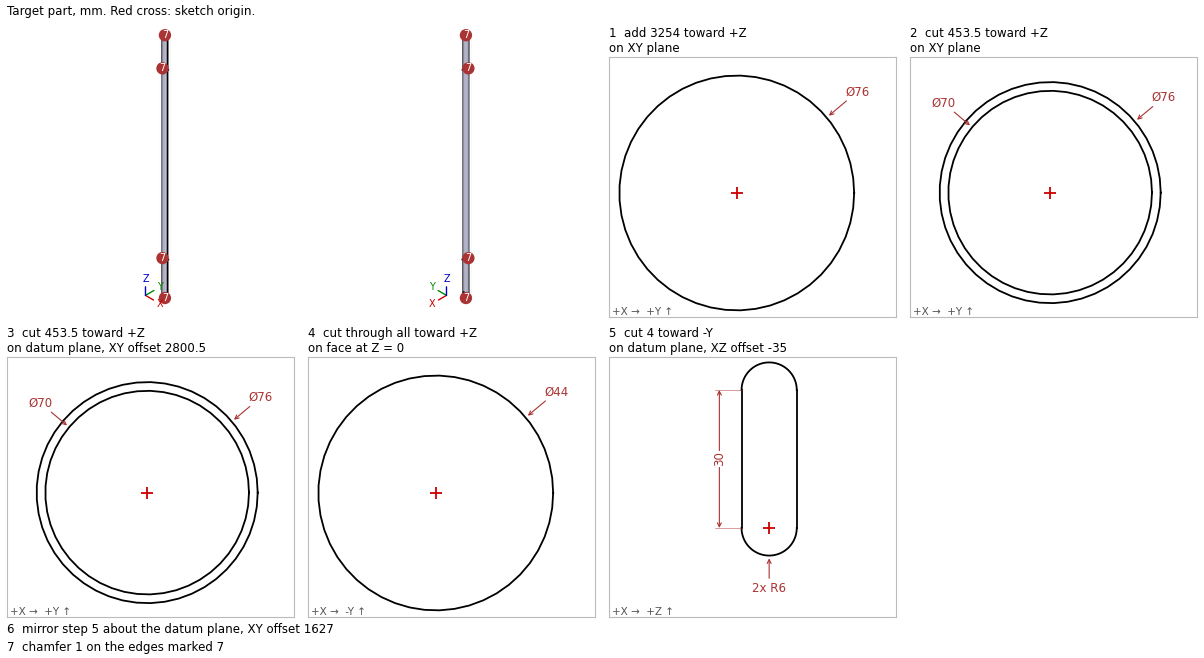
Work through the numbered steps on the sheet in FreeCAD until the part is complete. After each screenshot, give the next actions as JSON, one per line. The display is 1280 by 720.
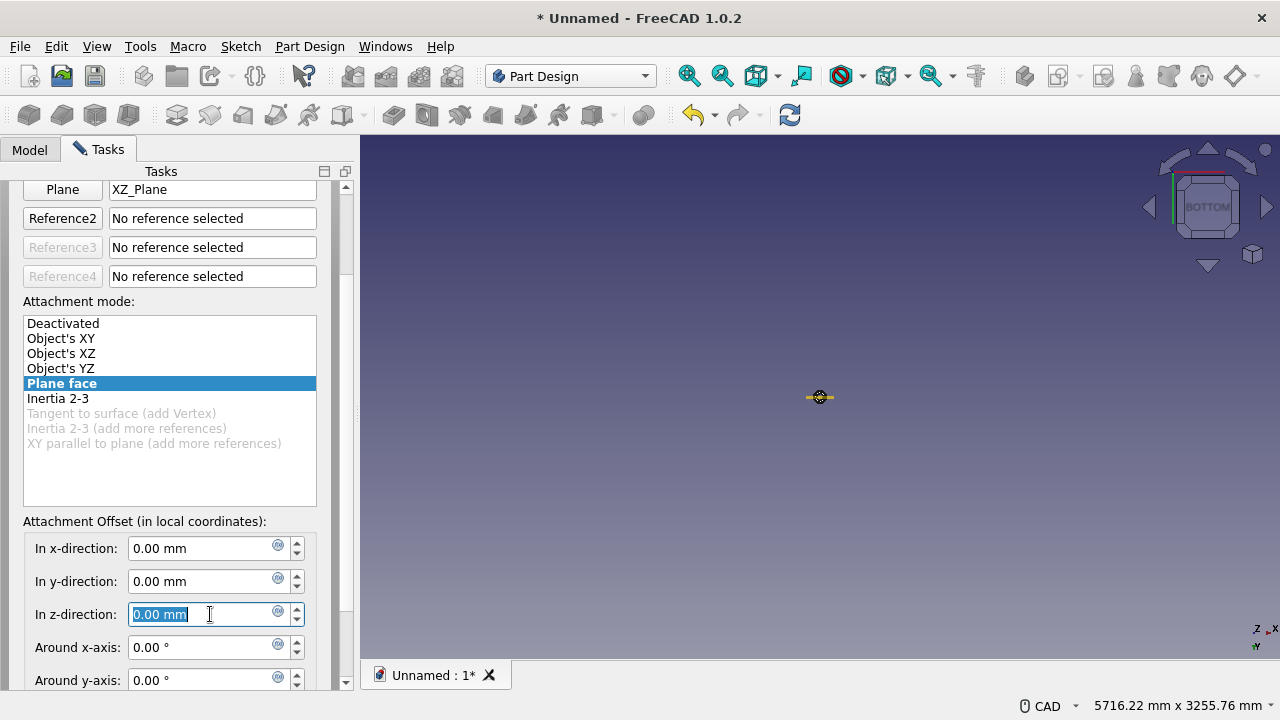
{"action": "type", "text": "-35"}
{"action": "key", "text": "Tab"}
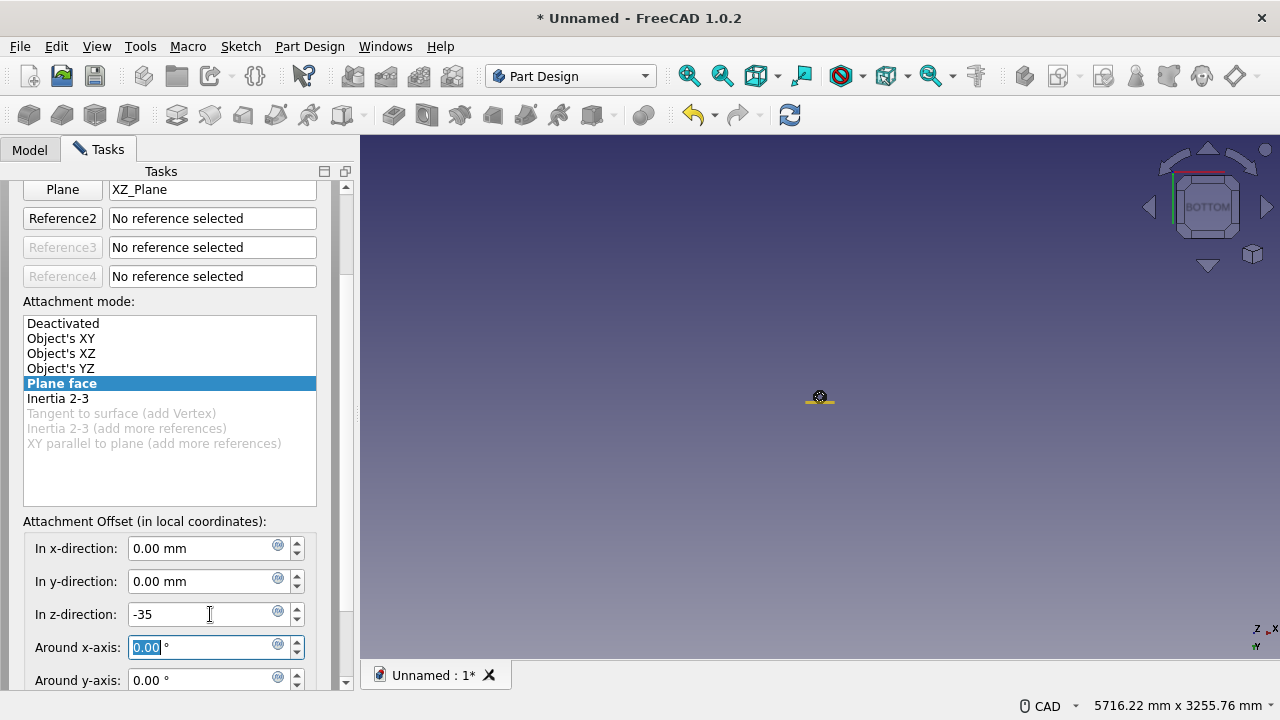
{"action": "scroll", "coordinate": [346, 436], "scroll_direction": "up", "scroll_amount": 3}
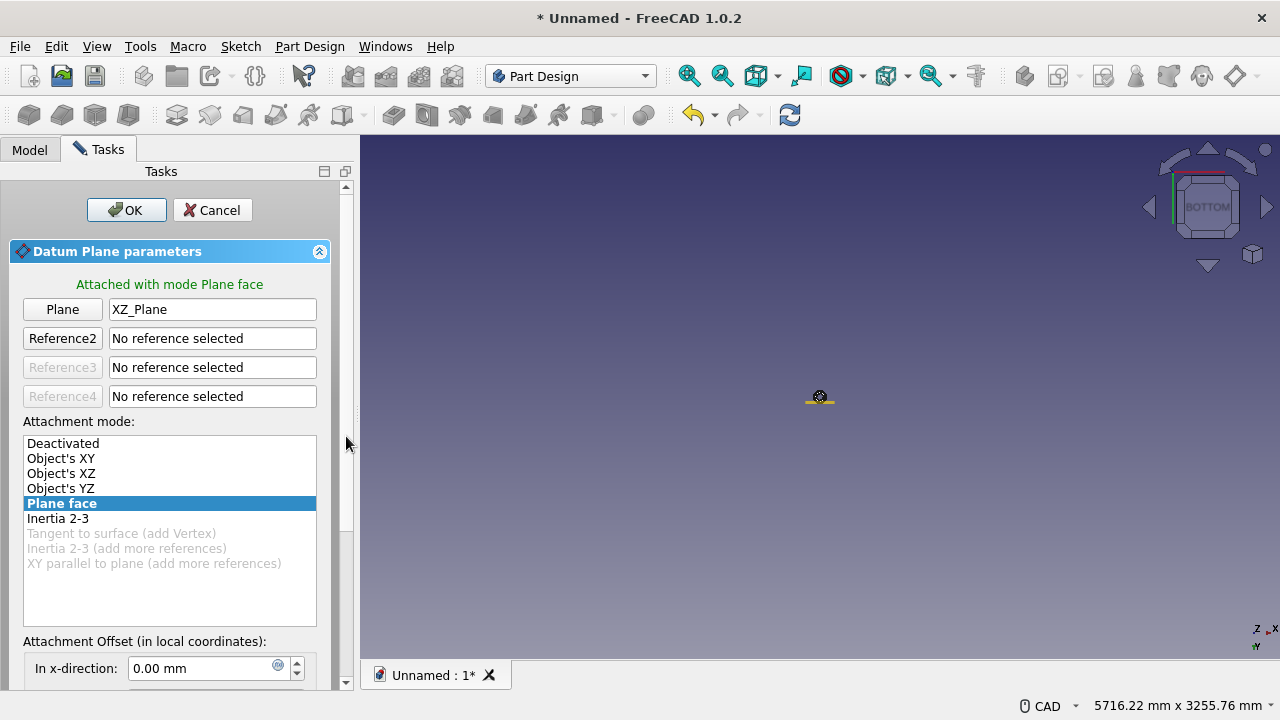
{"action": "left_click", "coordinate": [127, 210]}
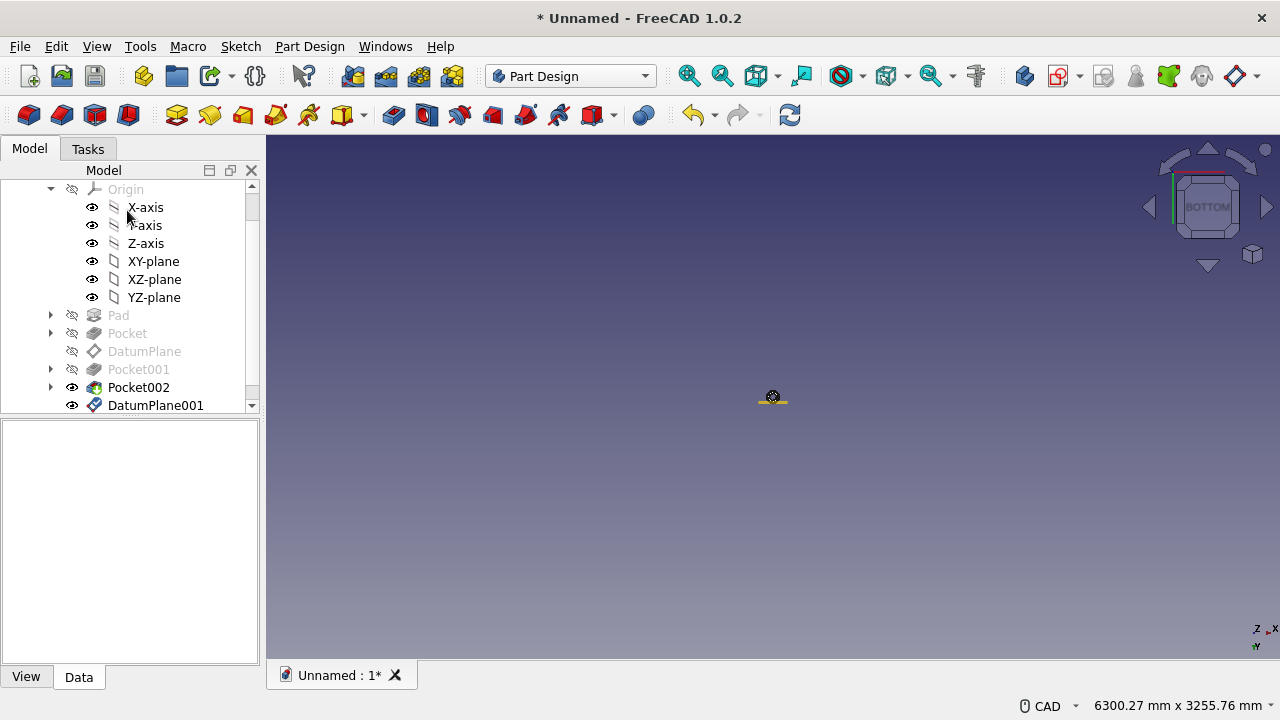
{"action": "left_click", "coordinate": [117, 405]}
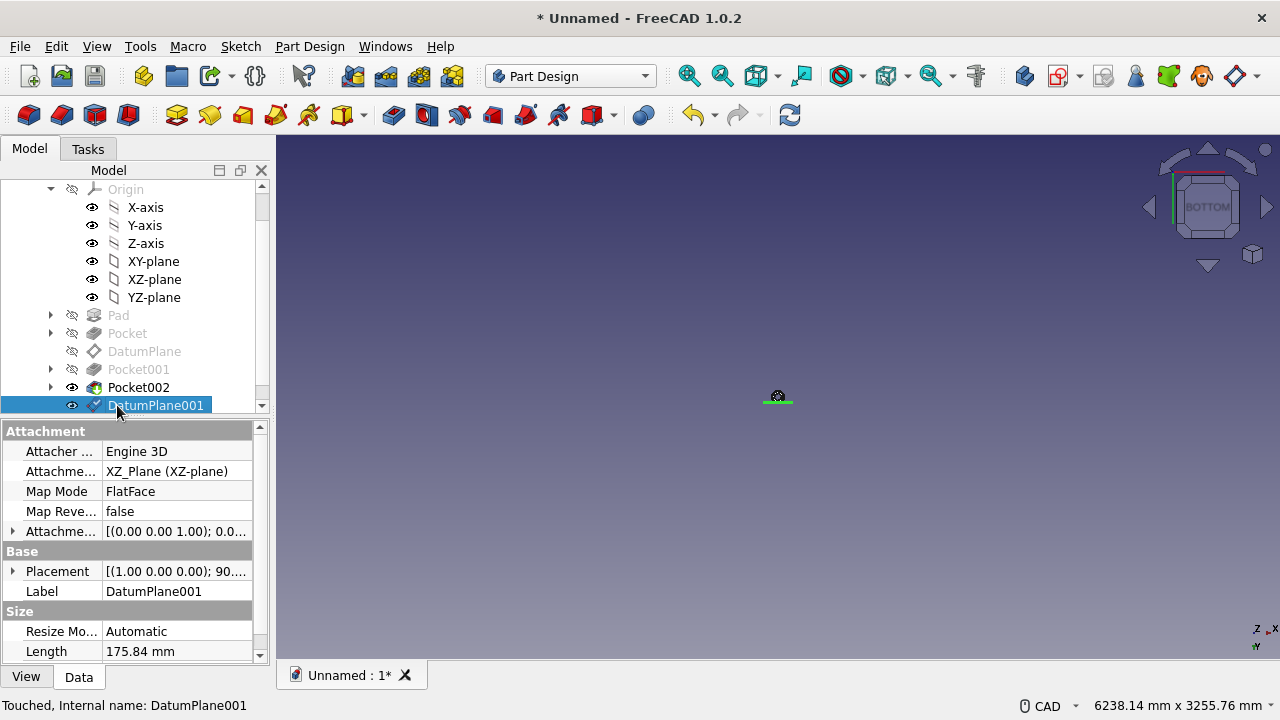
{"action": "left_click", "coordinate": [1058, 76]}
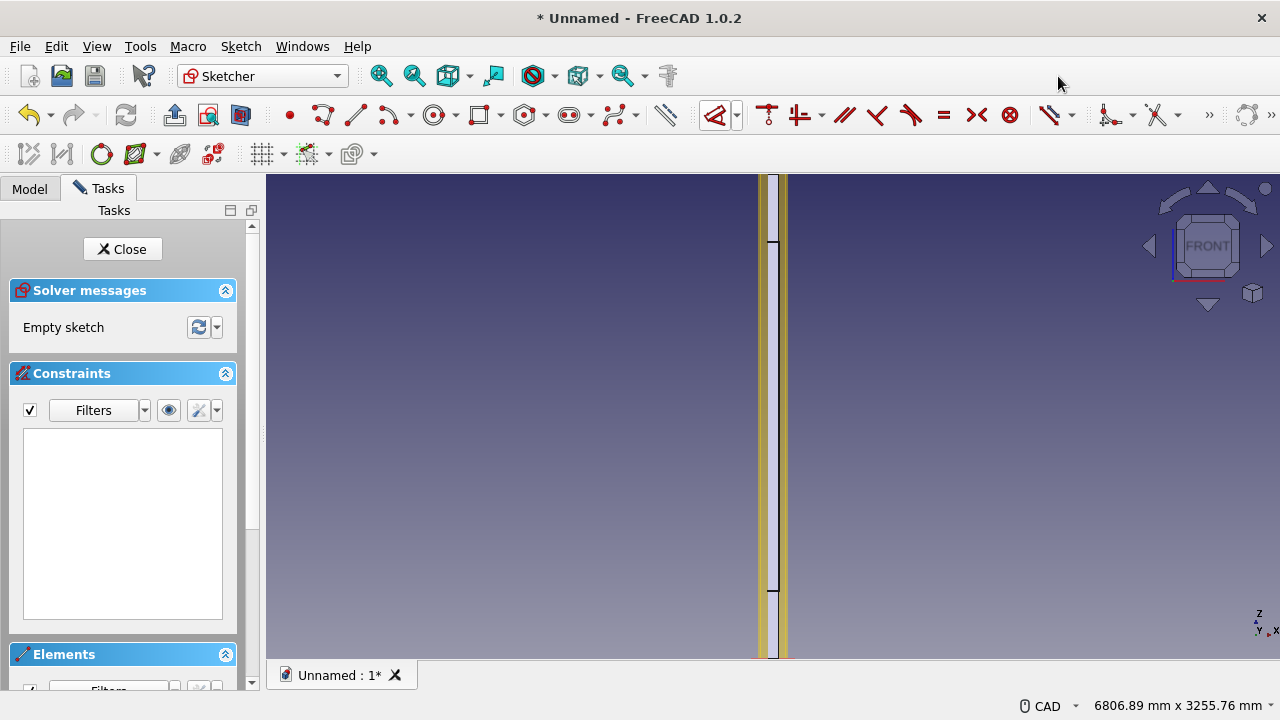
{"action": "left_click", "coordinate": [241, 116]}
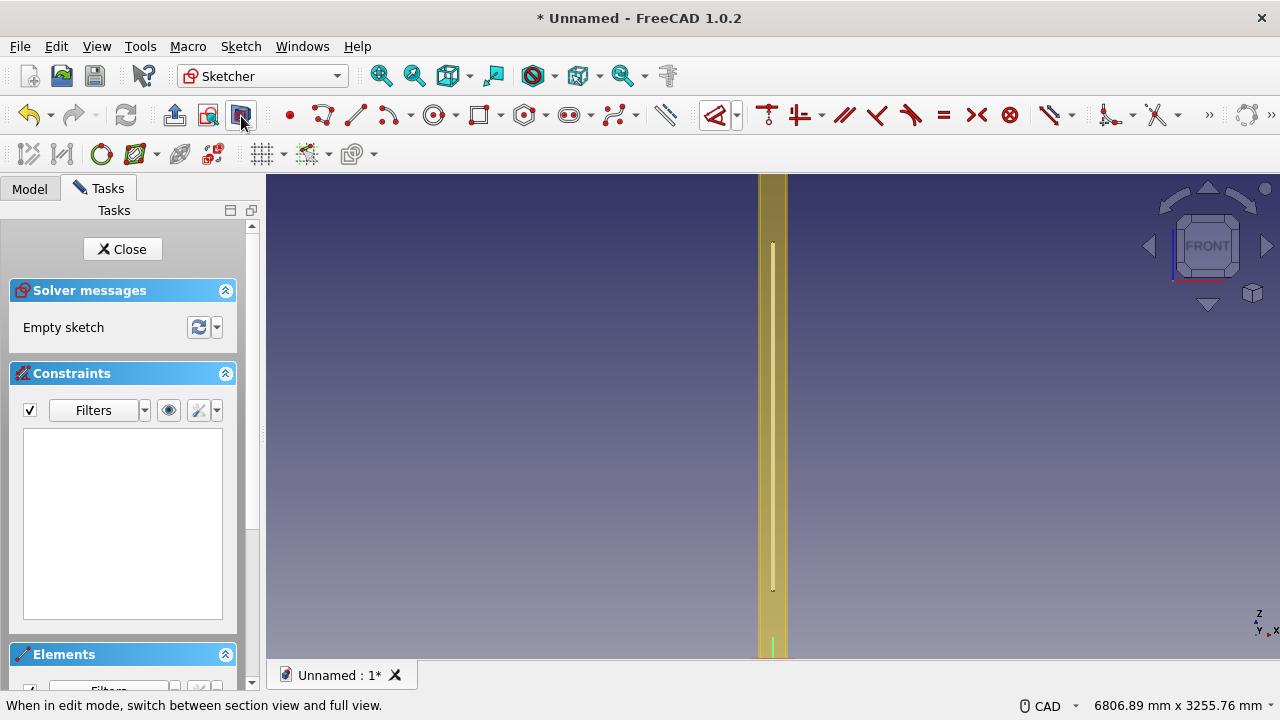
{"action": "scroll", "coordinate": [704, 416], "scroll_direction": "down", "scroll_amount": 5}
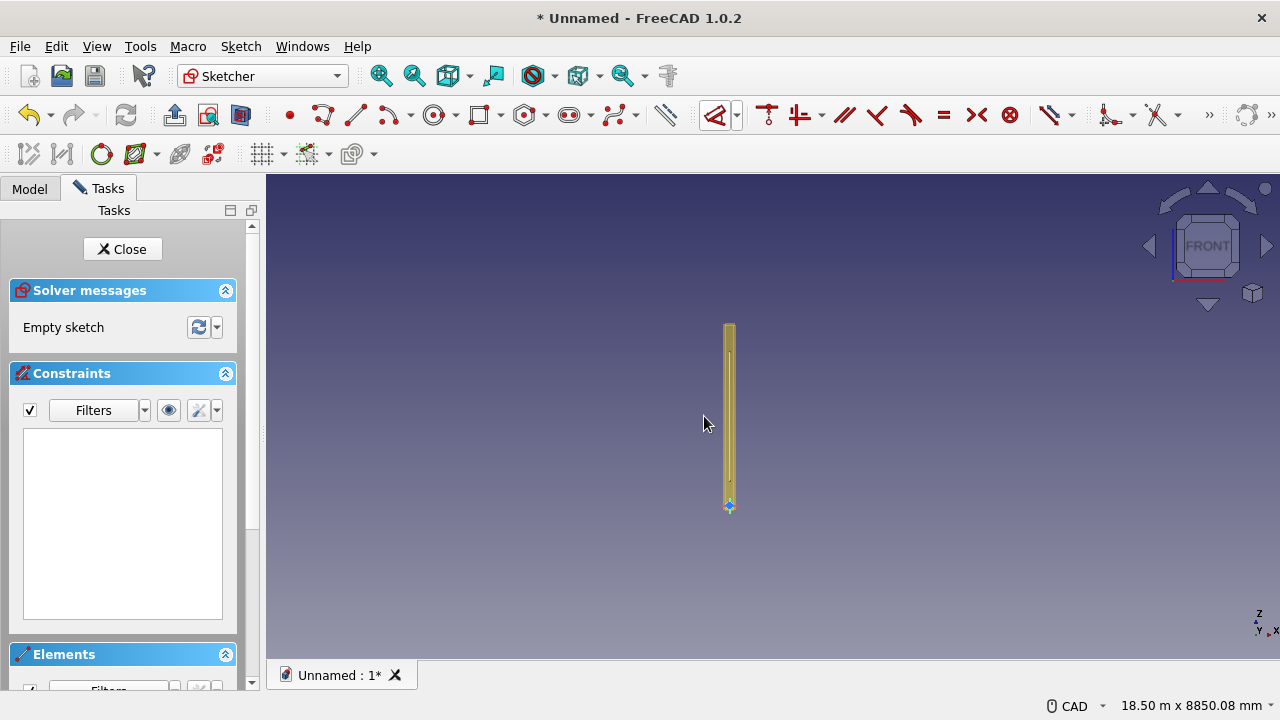
{"action": "scroll", "coordinate": [731, 509], "scroll_direction": "up", "scroll_amount": 15}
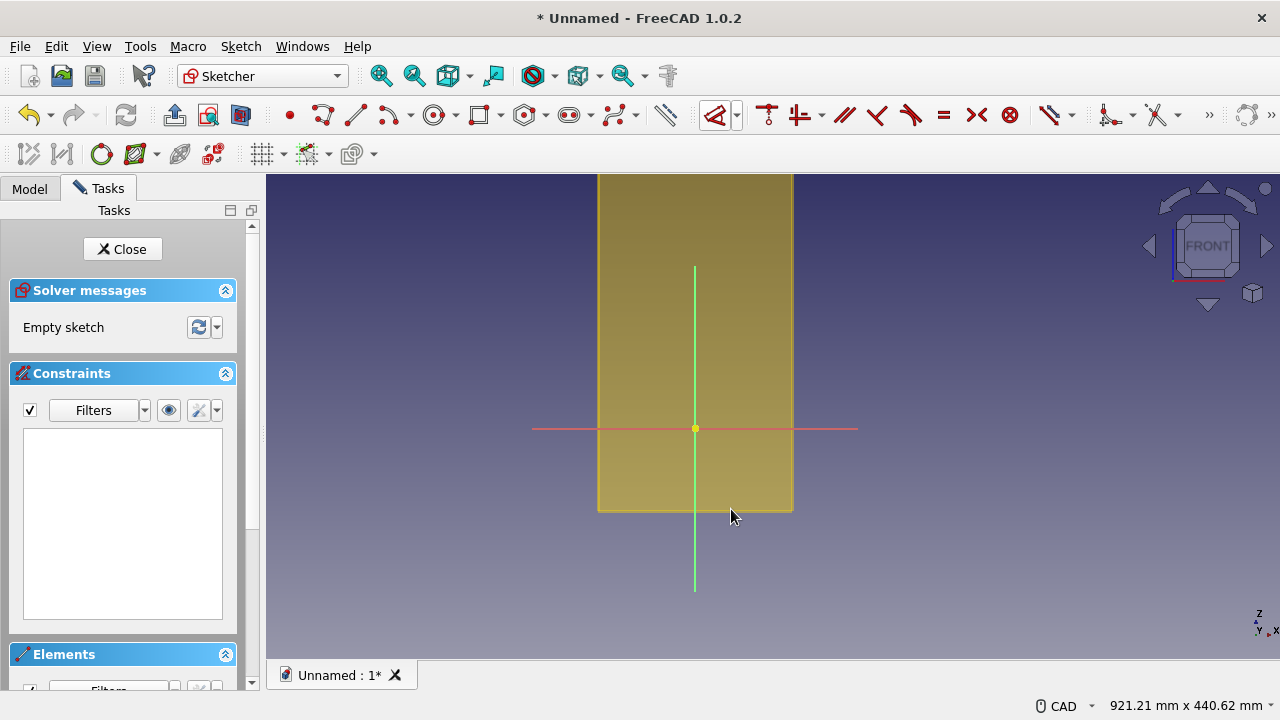
{"action": "scroll", "coordinate": [693, 411], "scroll_direction": "up", "scroll_amount": 9}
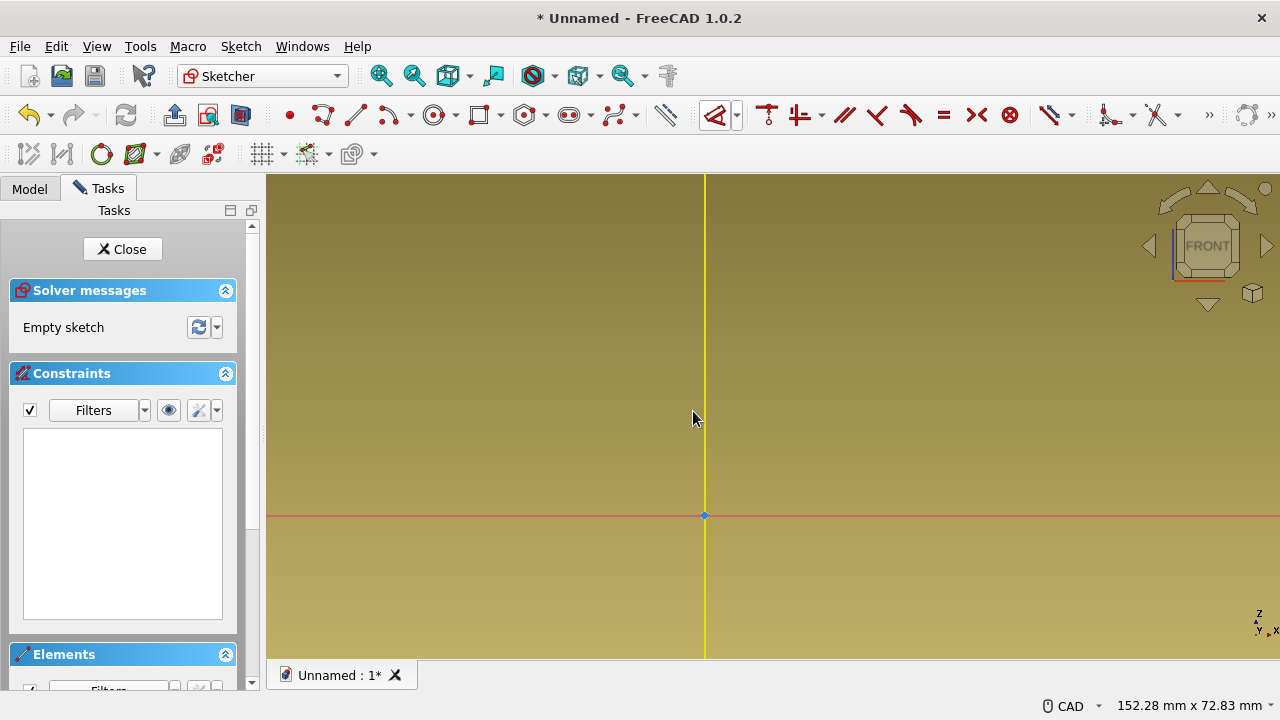
{"action": "left_click", "coordinate": [568, 116]}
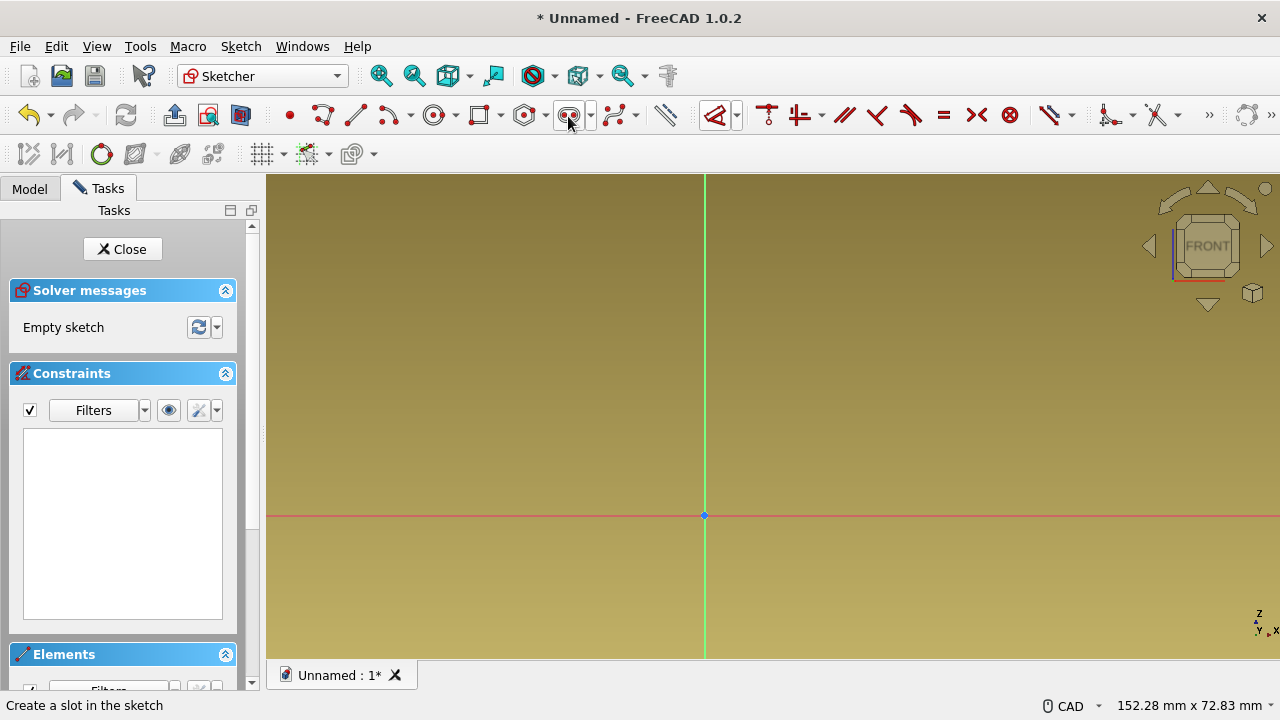
{"action": "left_click", "coordinate": [705, 516]}